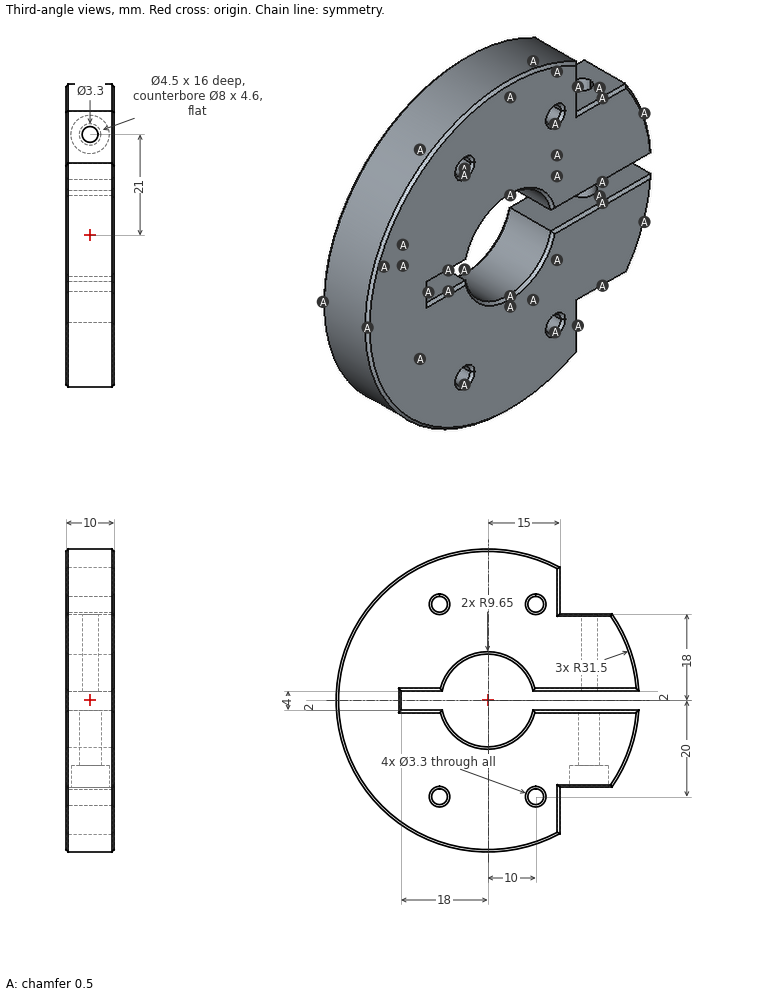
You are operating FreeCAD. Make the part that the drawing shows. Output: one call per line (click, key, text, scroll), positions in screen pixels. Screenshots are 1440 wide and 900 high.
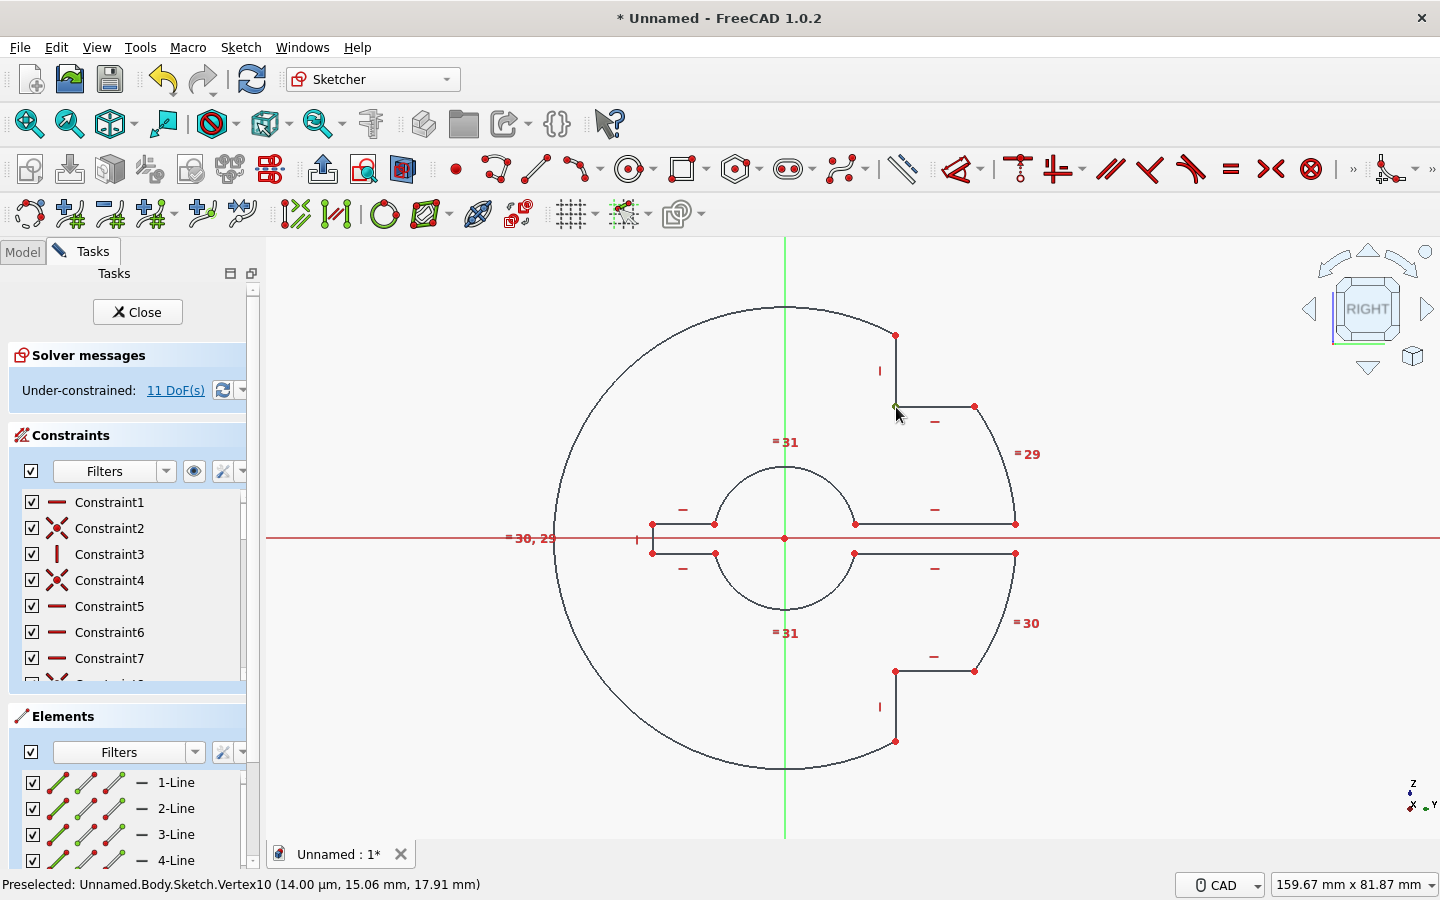
click(896, 671)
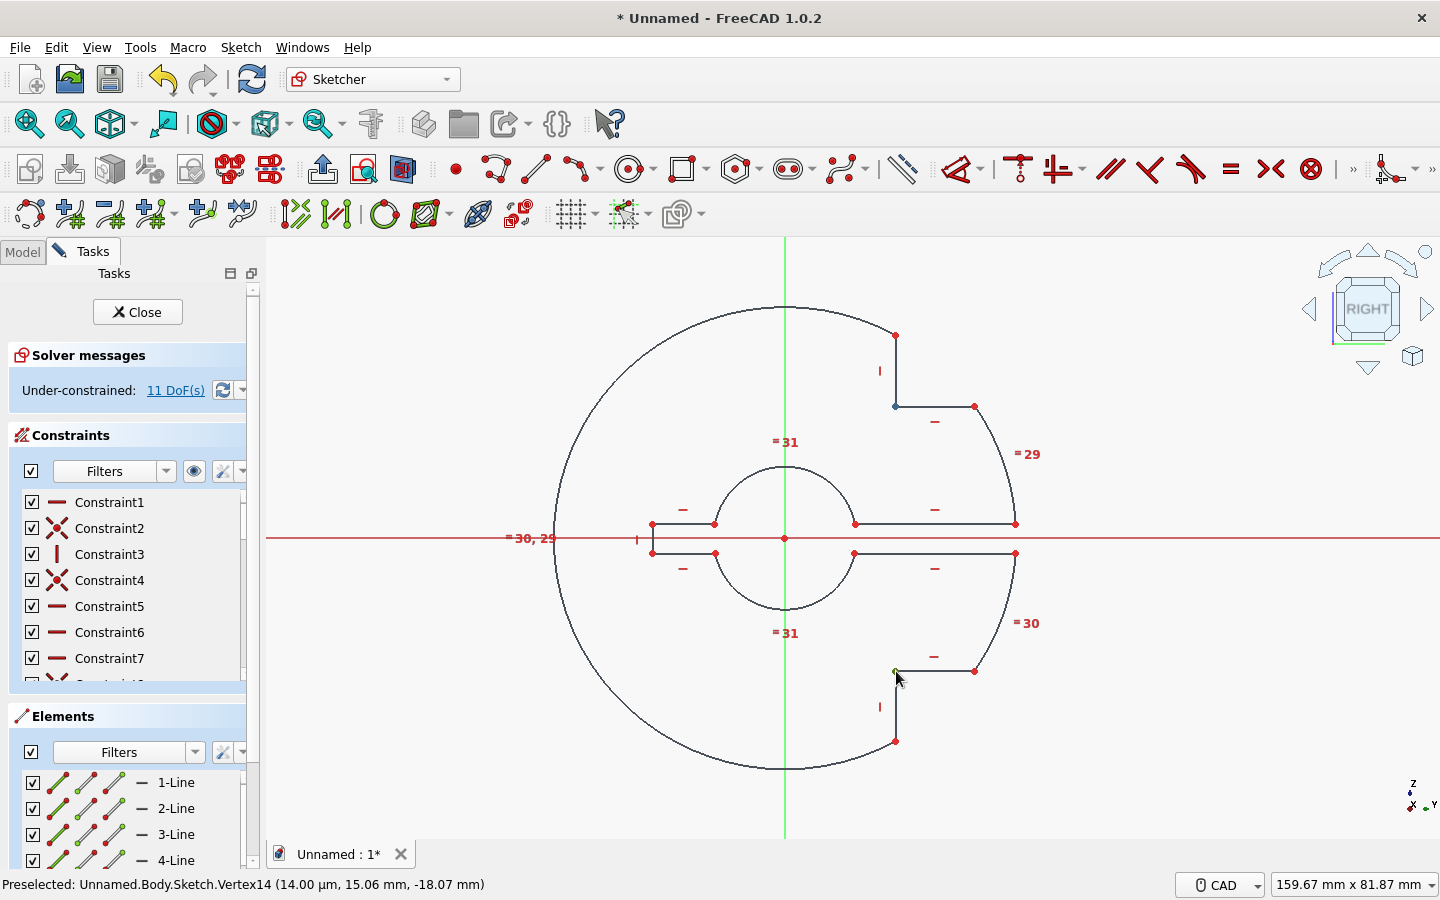
click(364, 538)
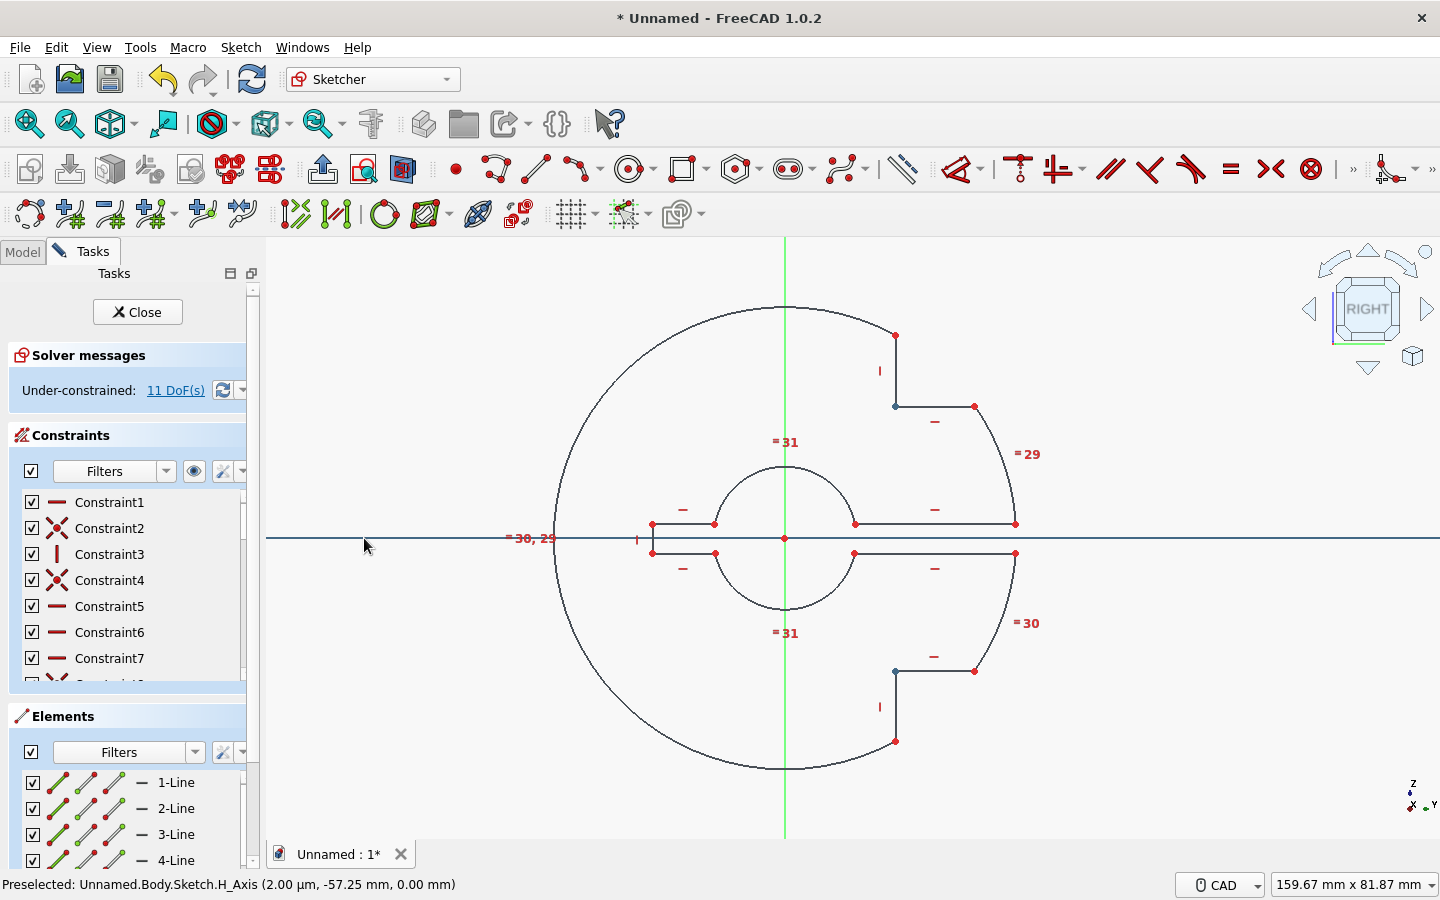
key(s)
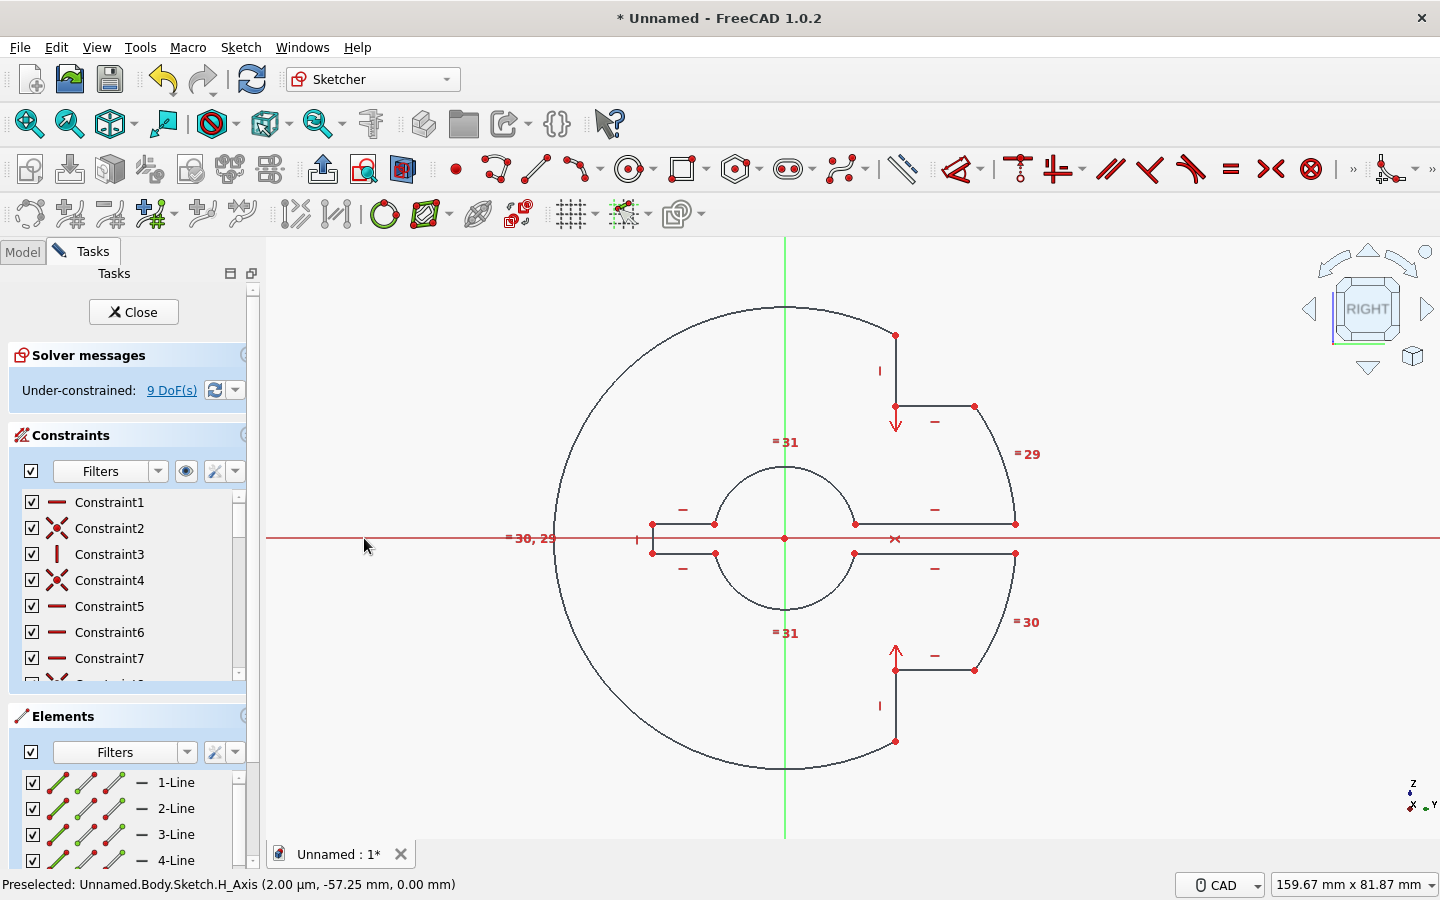
click(956, 170)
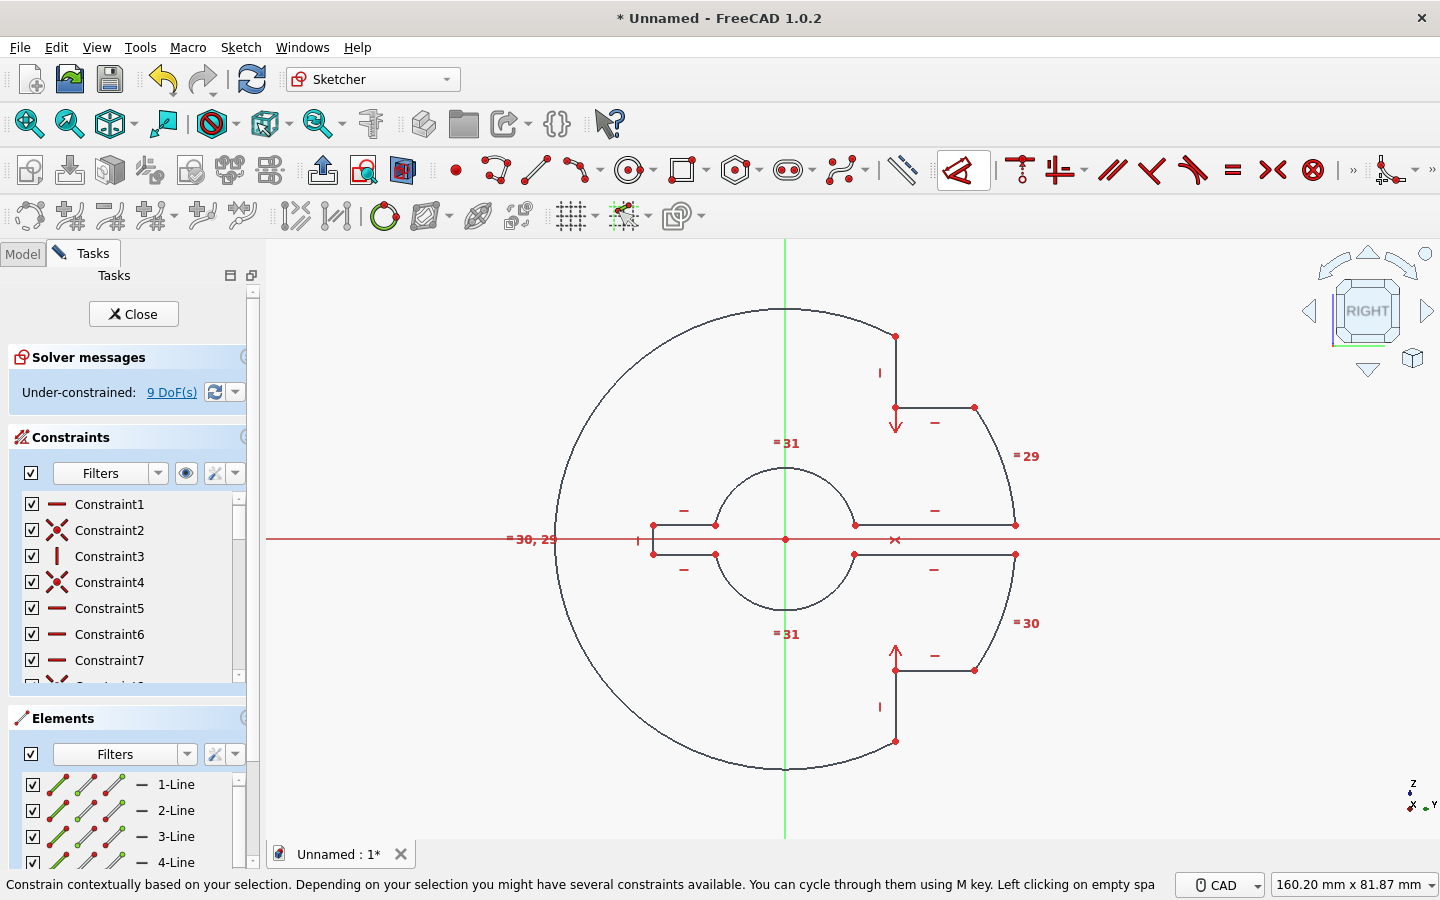
click(822, 479)
click(839, 452)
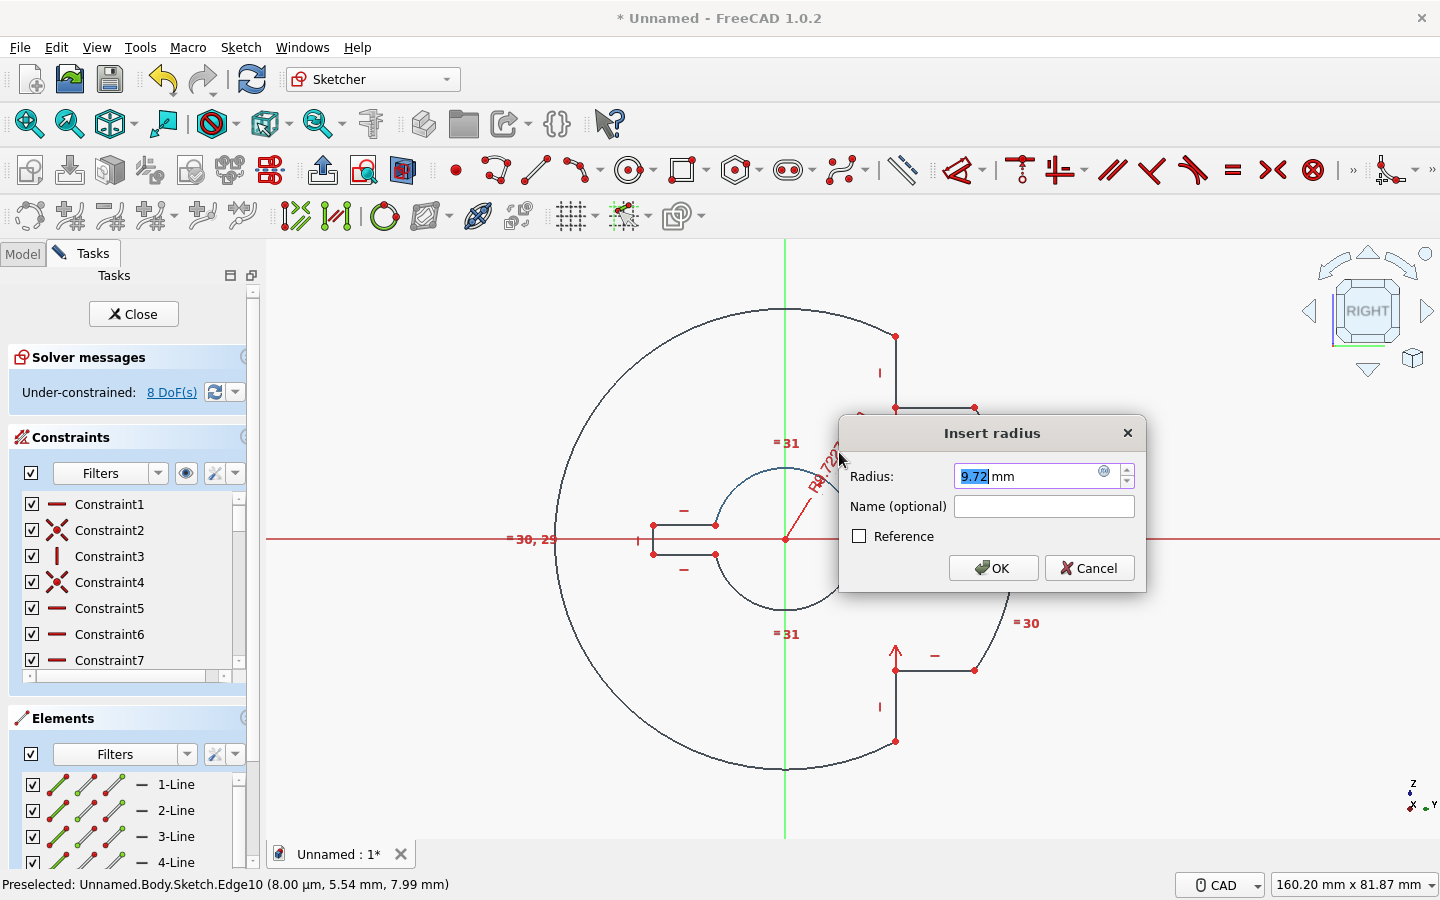
text(9.65)
key(Return)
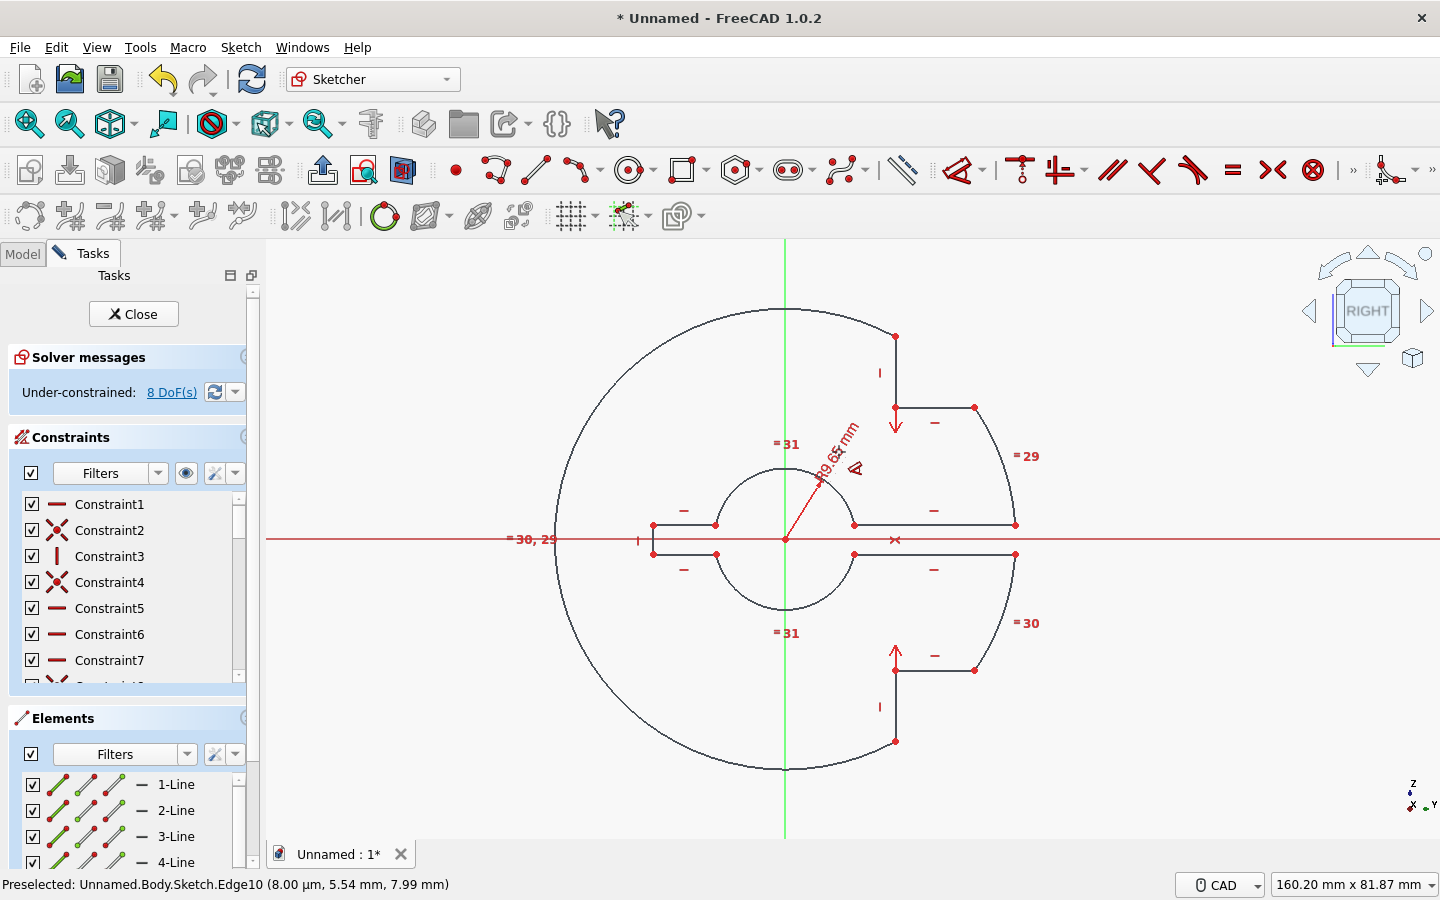
click(1010, 488)
click(1041, 481)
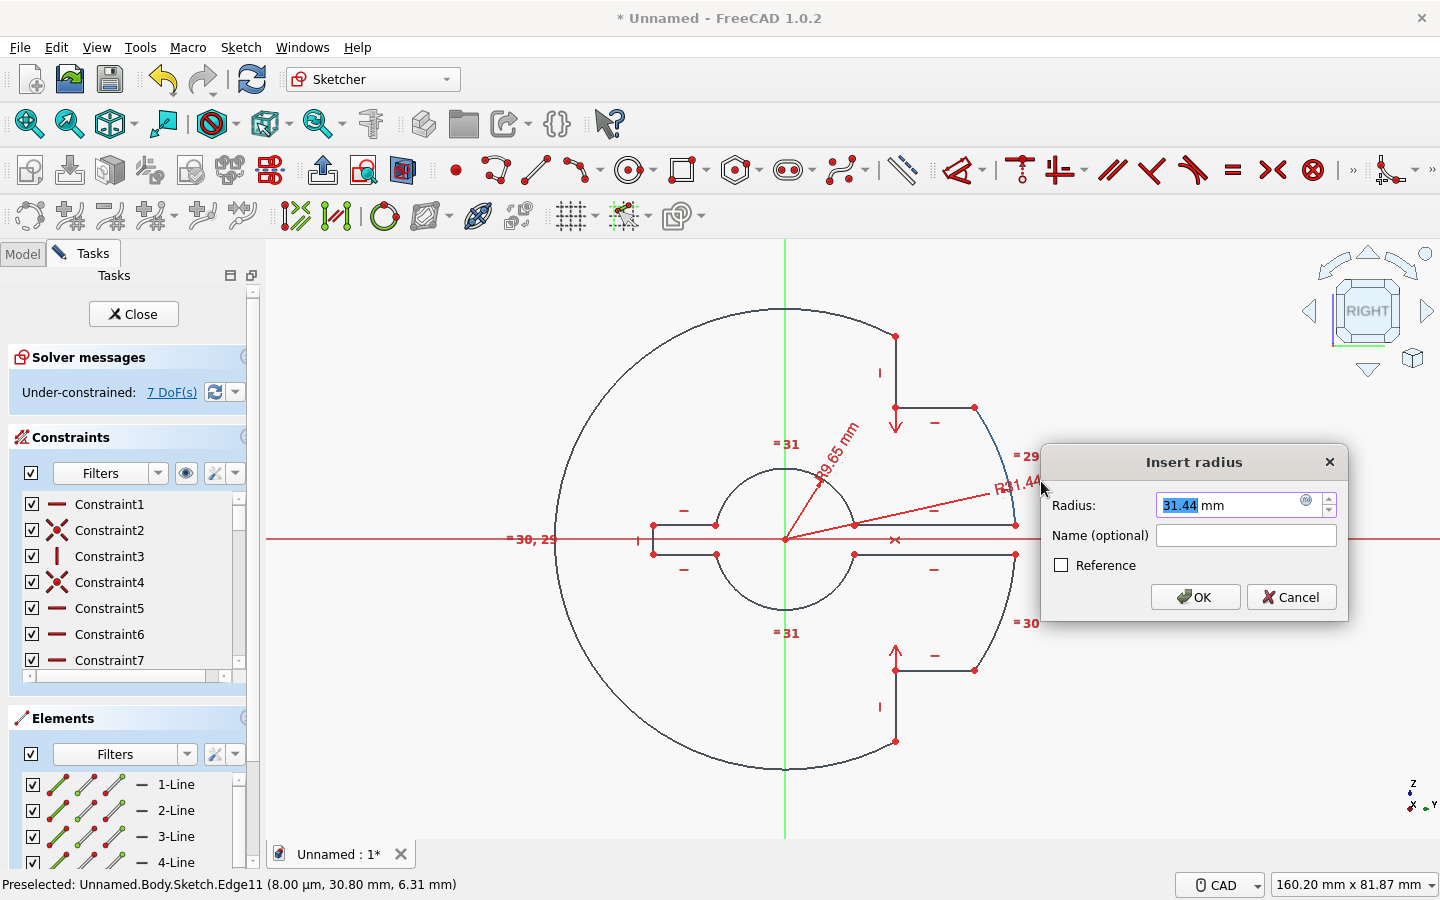
text(31.5)
key(Return)